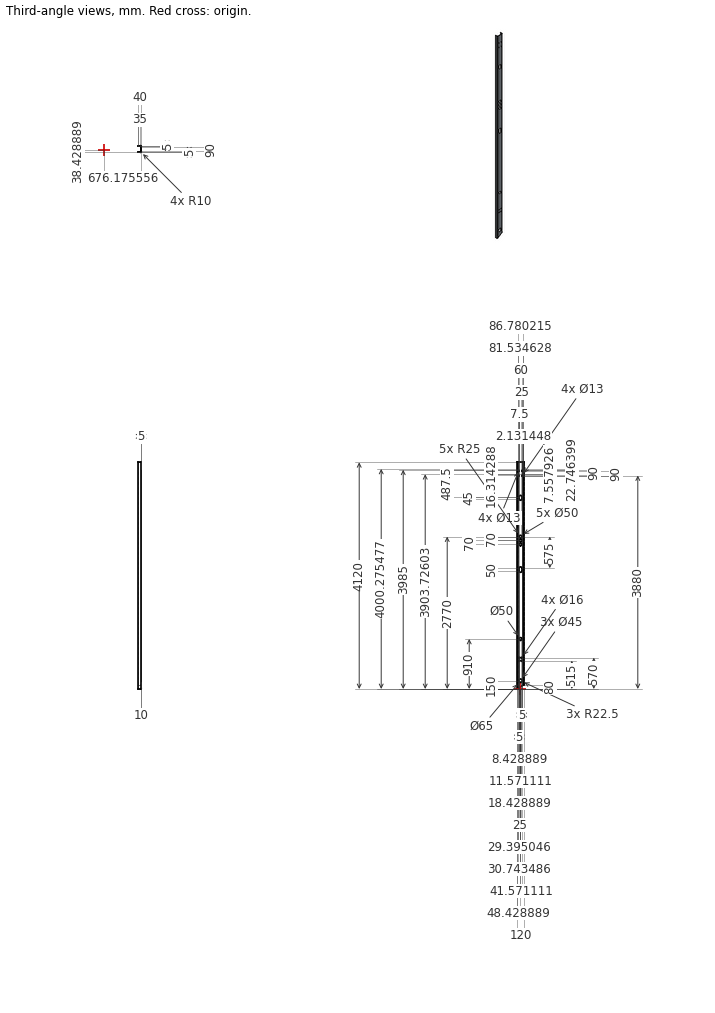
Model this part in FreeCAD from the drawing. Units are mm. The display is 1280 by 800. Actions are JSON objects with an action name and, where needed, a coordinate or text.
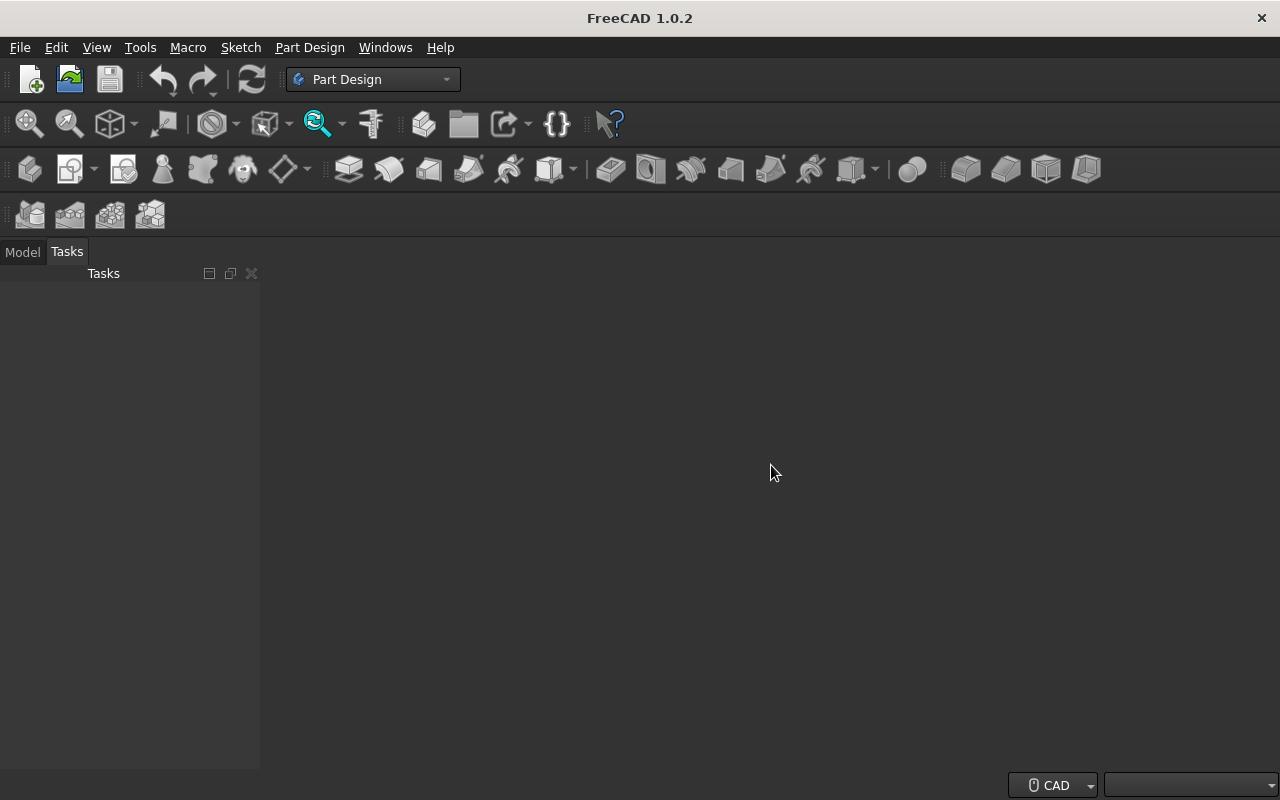
{"action": "key", "text": "ctrl+n"}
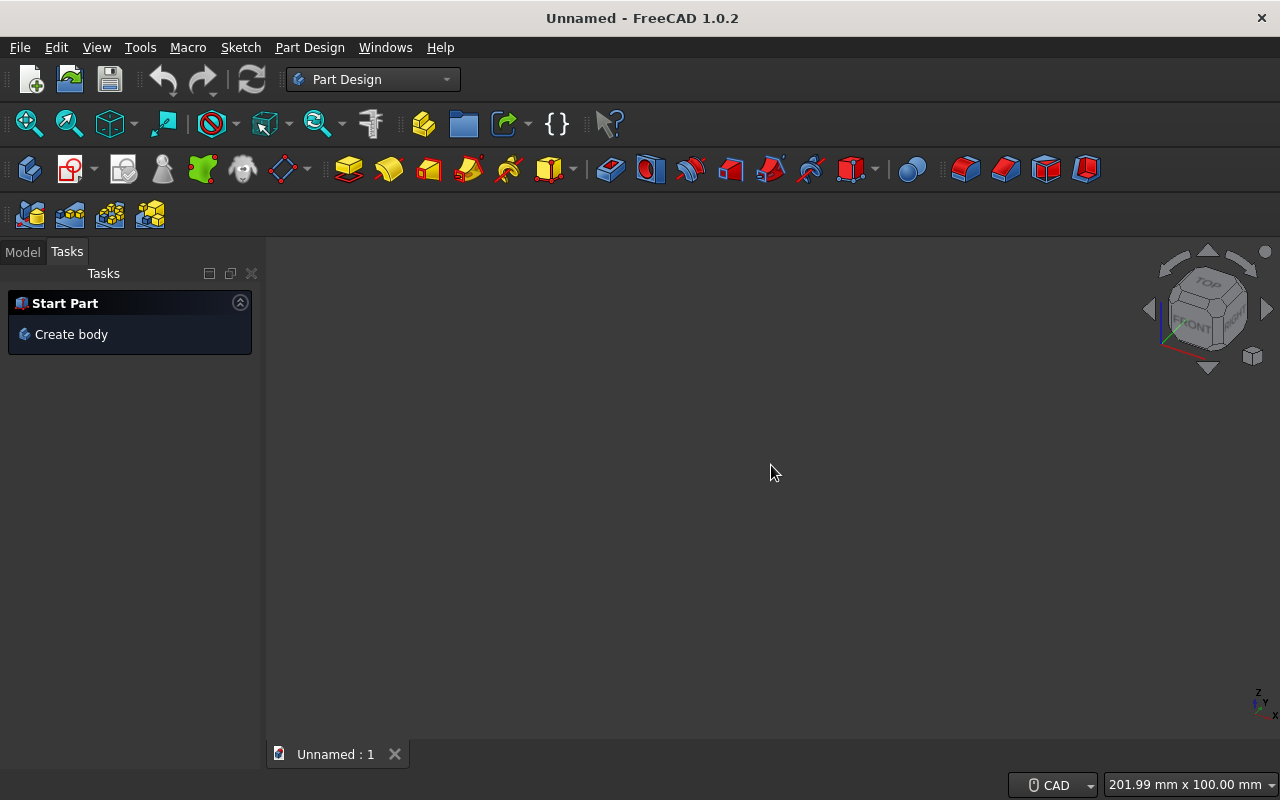
{"action": "left_click", "coordinate": [70, 170]}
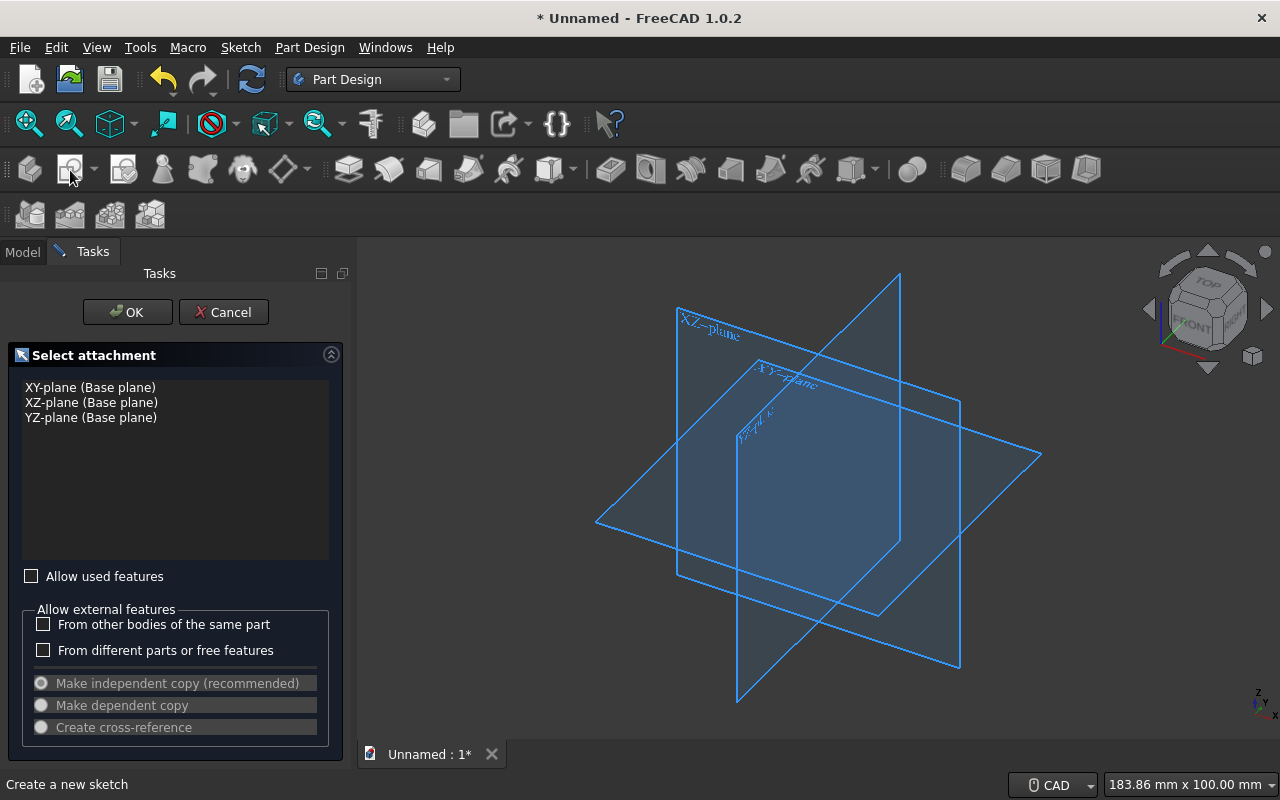
{"action": "left_click", "coordinate": [82, 388]}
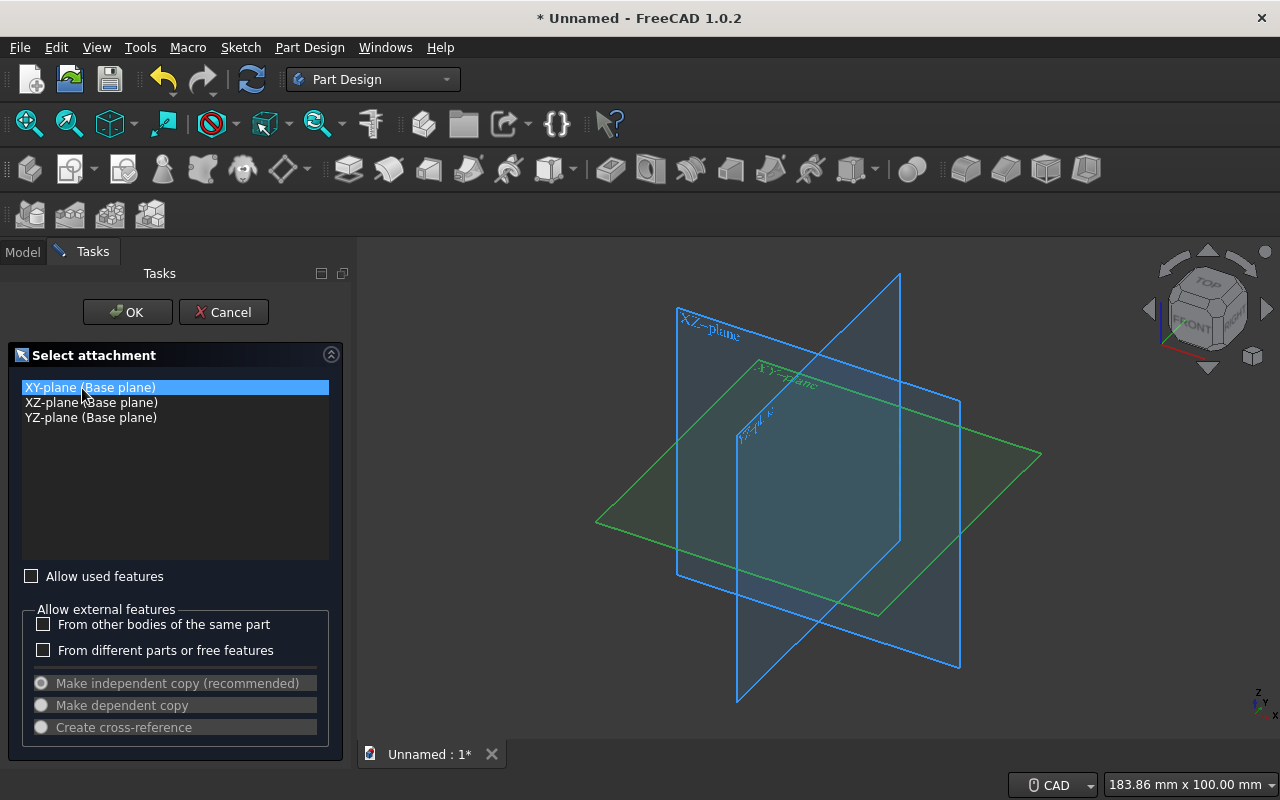
{"action": "left_click", "coordinate": [128, 312]}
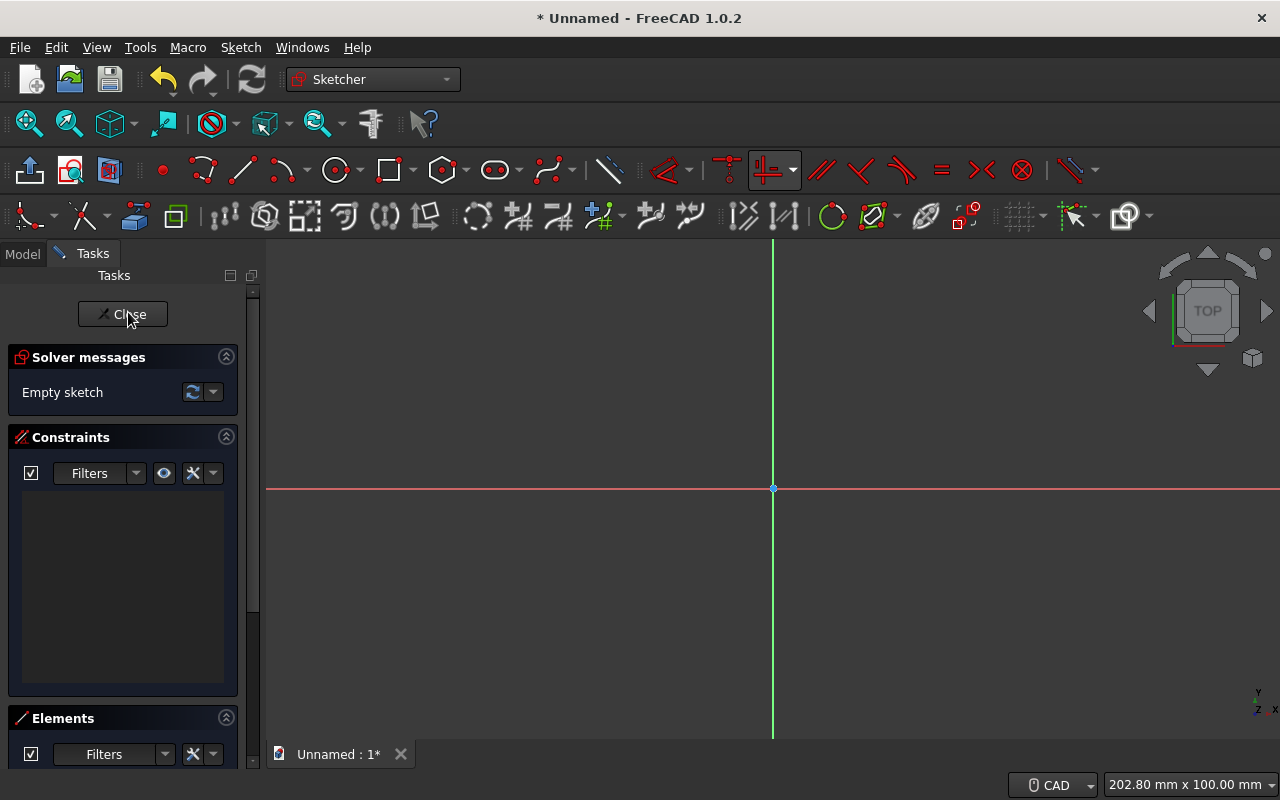
{"action": "scroll", "coordinate": [704, 489], "scroll_direction": "down", "scroll_amount": 5}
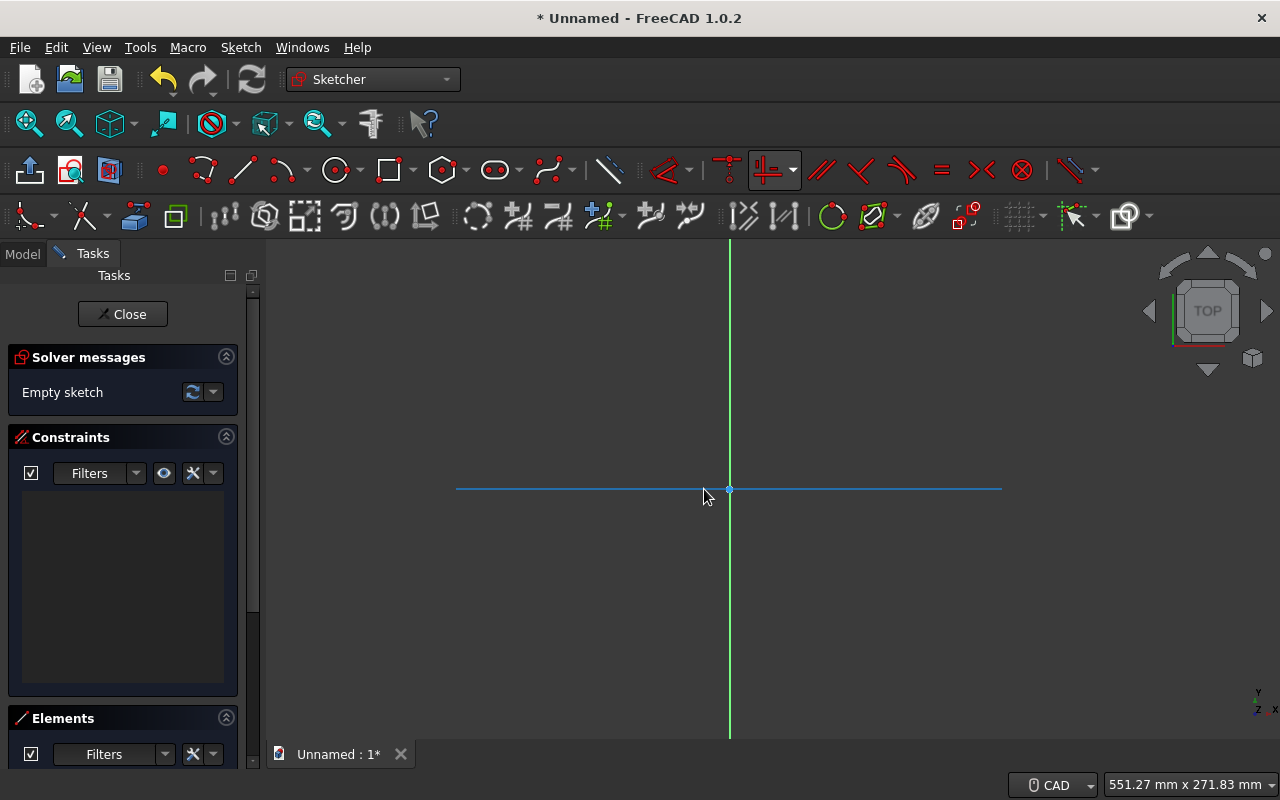
{"action": "scroll", "coordinate": [704, 489], "scroll_direction": "down", "scroll_amount": 5}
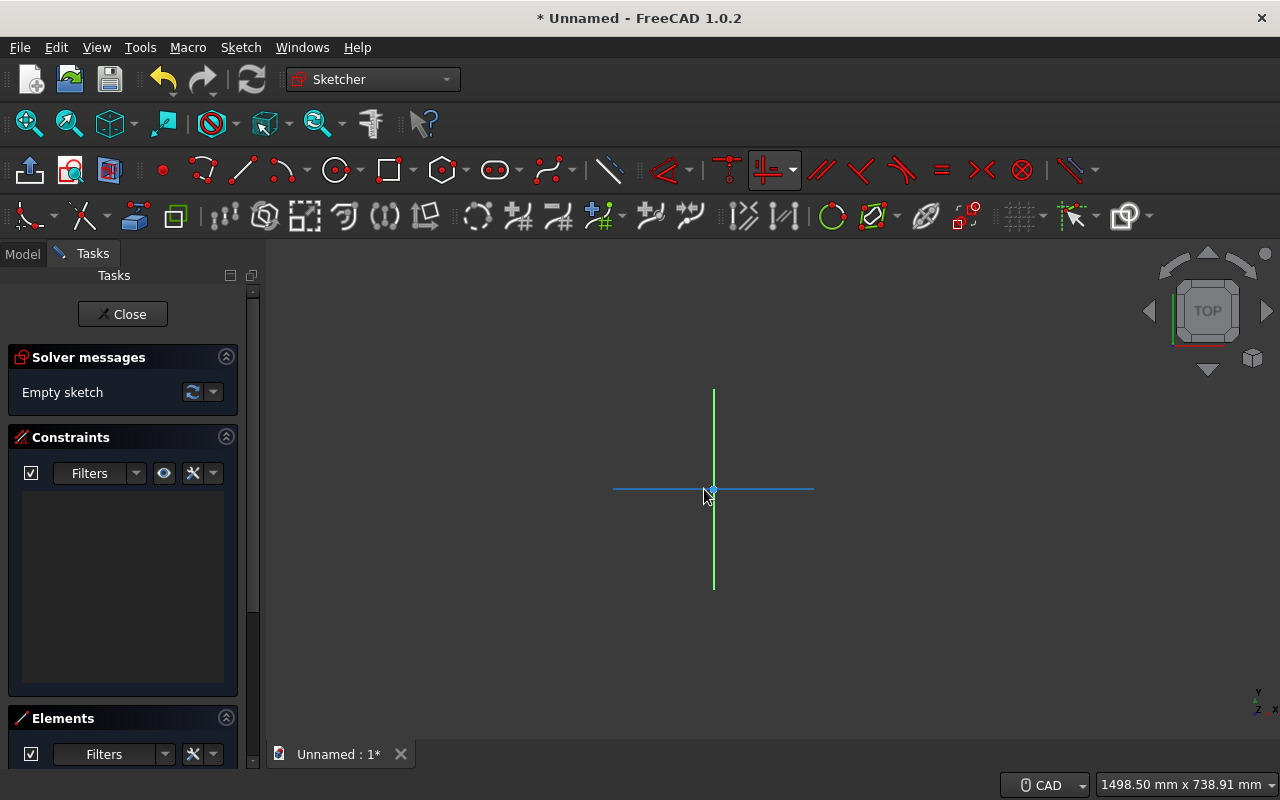
{"action": "scroll", "coordinate": [704, 489], "scroll_direction": "down", "scroll_amount": 5}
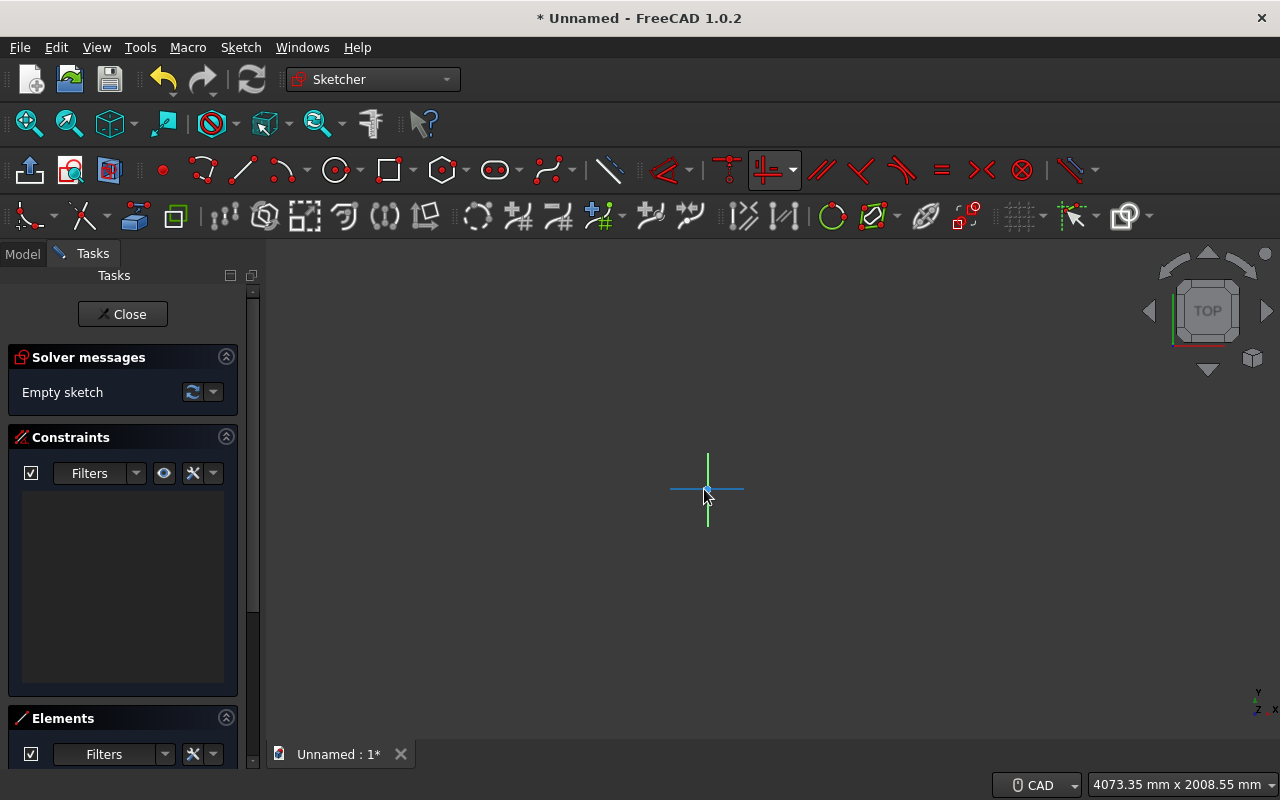
{"action": "scroll", "coordinate": [886, 486], "scroll_direction": "up", "scroll_amount": 12}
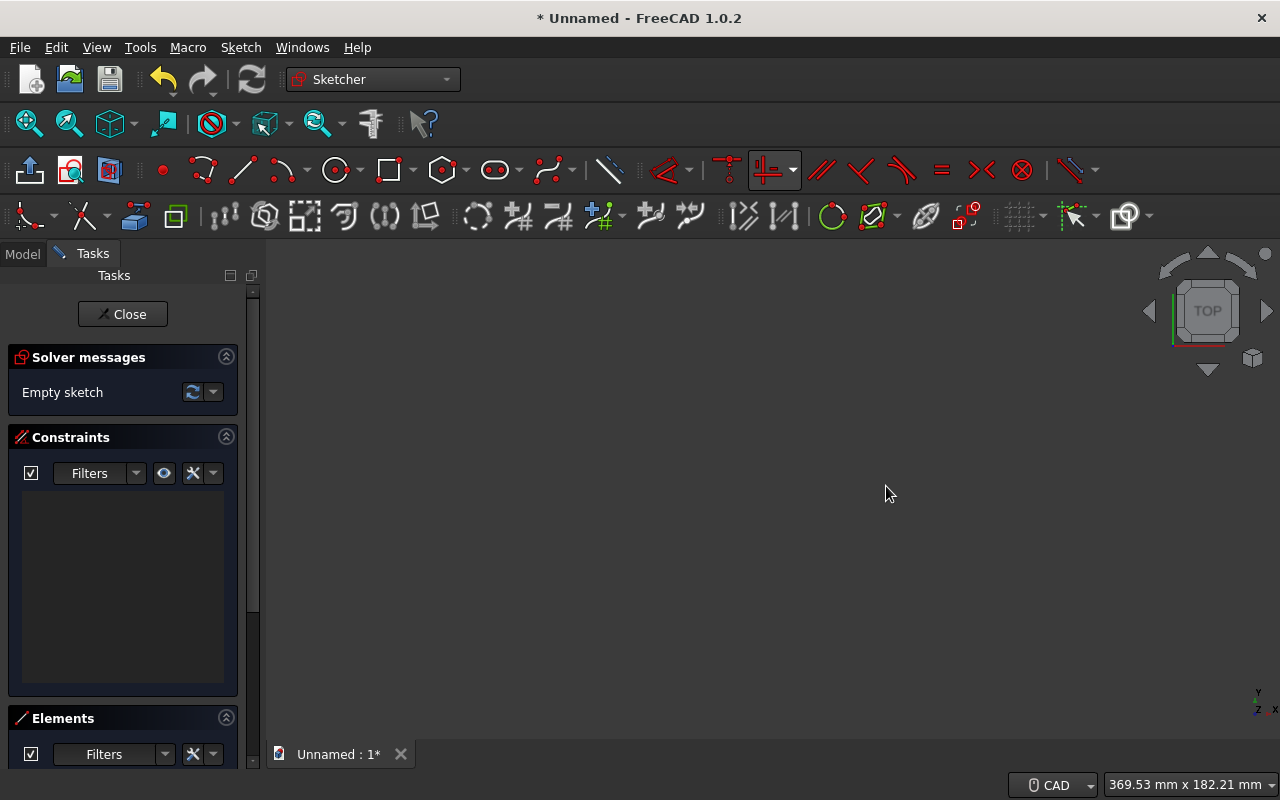
{"action": "left_click", "coordinate": [244, 170]}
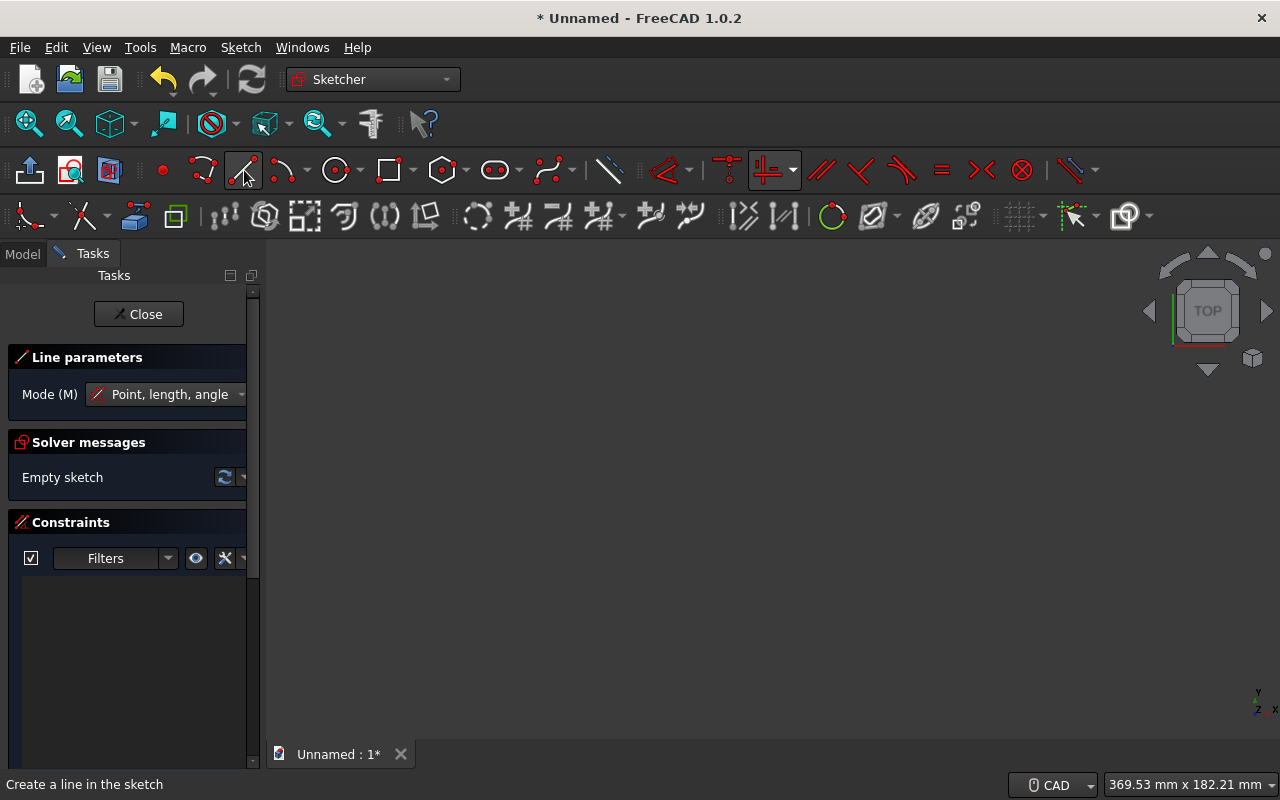
{"action": "left_click", "coordinate": [772, 625]}
{"action": "left_click", "coordinate": [772, 350]}